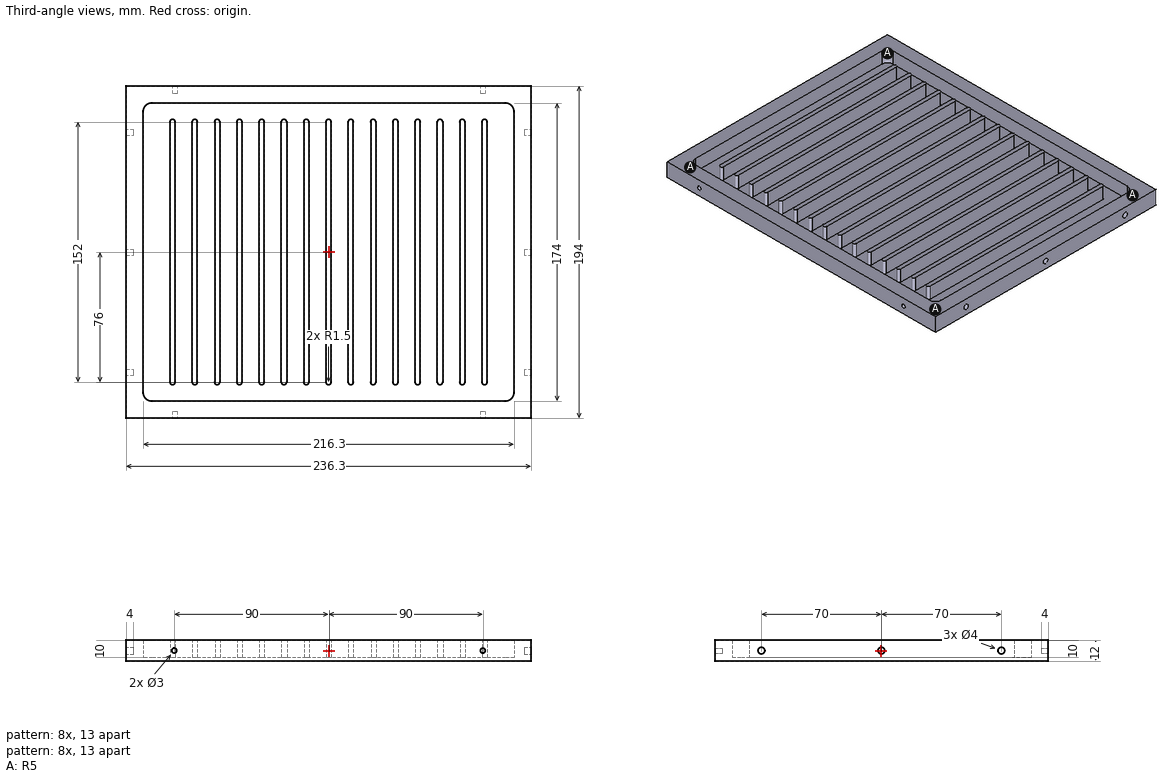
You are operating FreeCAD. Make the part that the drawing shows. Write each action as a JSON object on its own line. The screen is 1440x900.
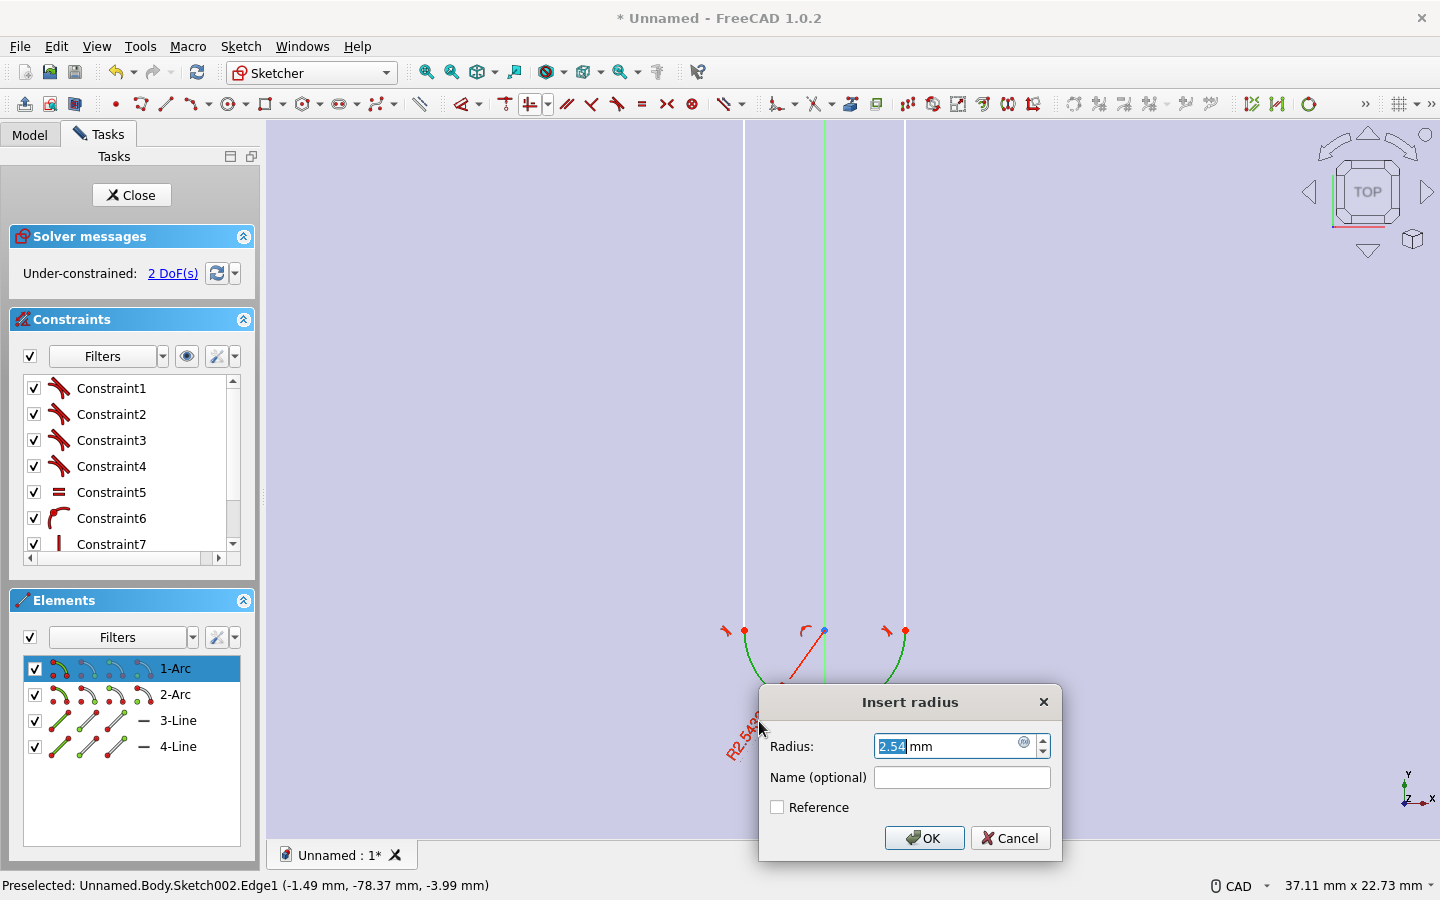
{"action": "type", "text": "1.5"}
{"action": "key", "text": "Return"}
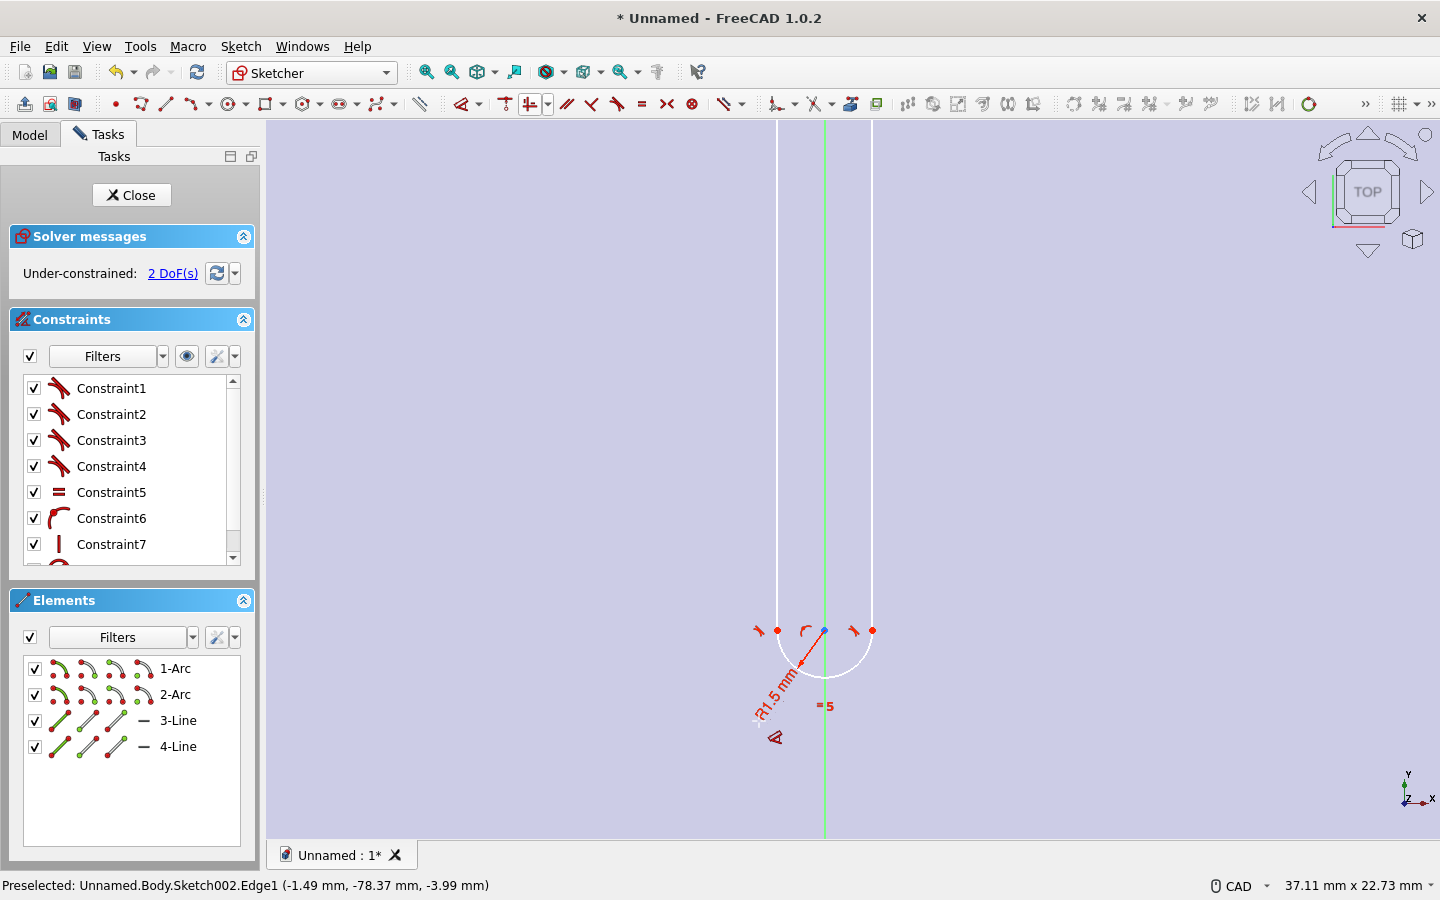
{"action": "scroll", "coordinate": [780, 705], "scroll_direction": "down", "scroll_amount": 12}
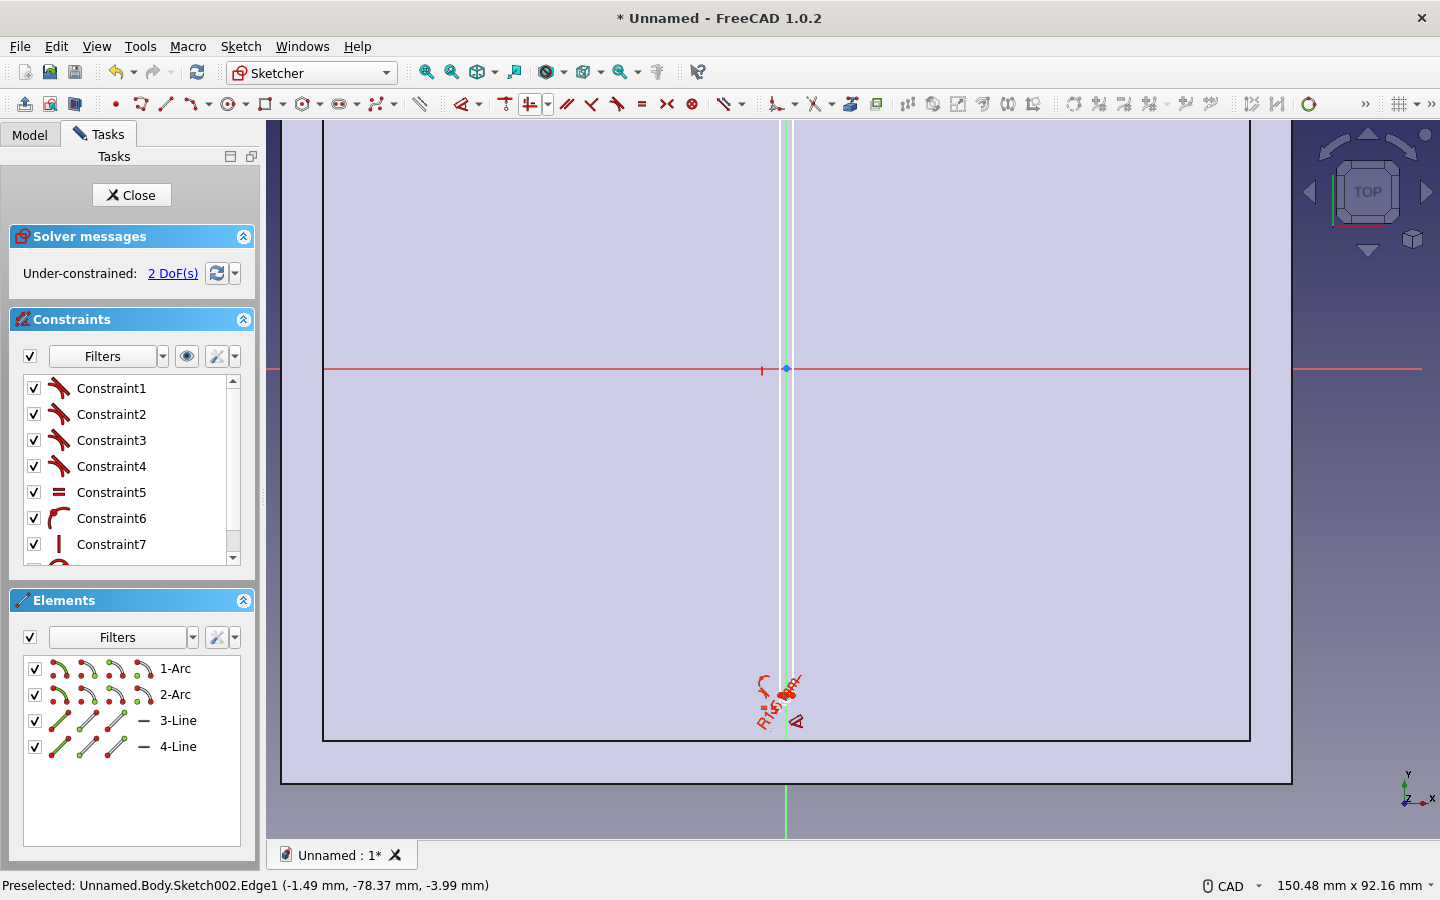
{"action": "scroll", "coordinate": [780, 568], "scroll_direction": "up", "scroll_amount": 6}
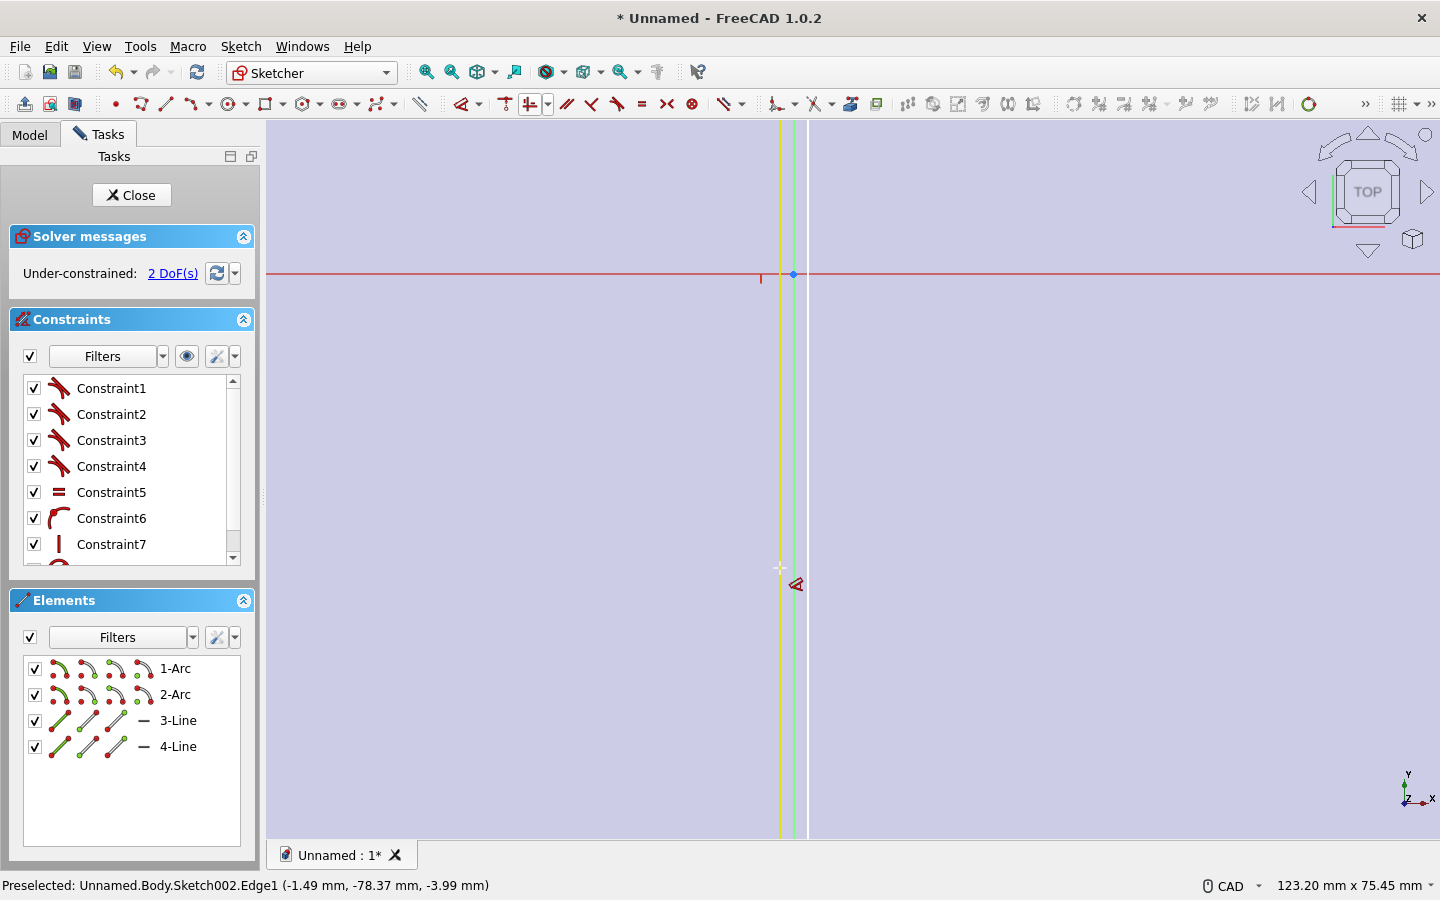
{"action": "left_click", "coordinate": [780, 567]}
{"action": "left_click", "coordinate": [746, 480]}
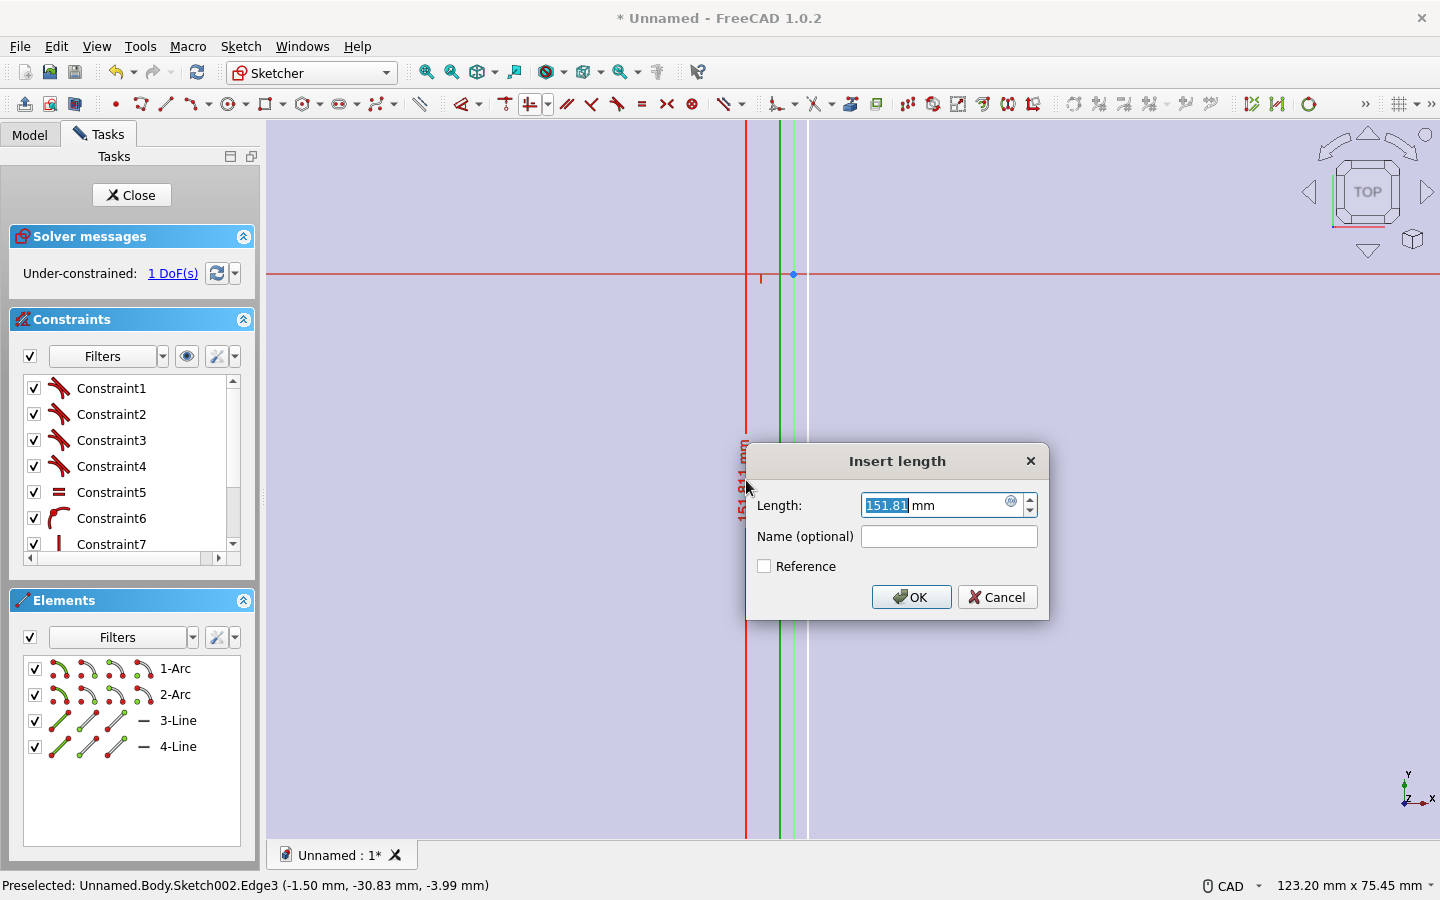
{"action": "type", "text": "152"}
{"action": "key", "text": "Return"}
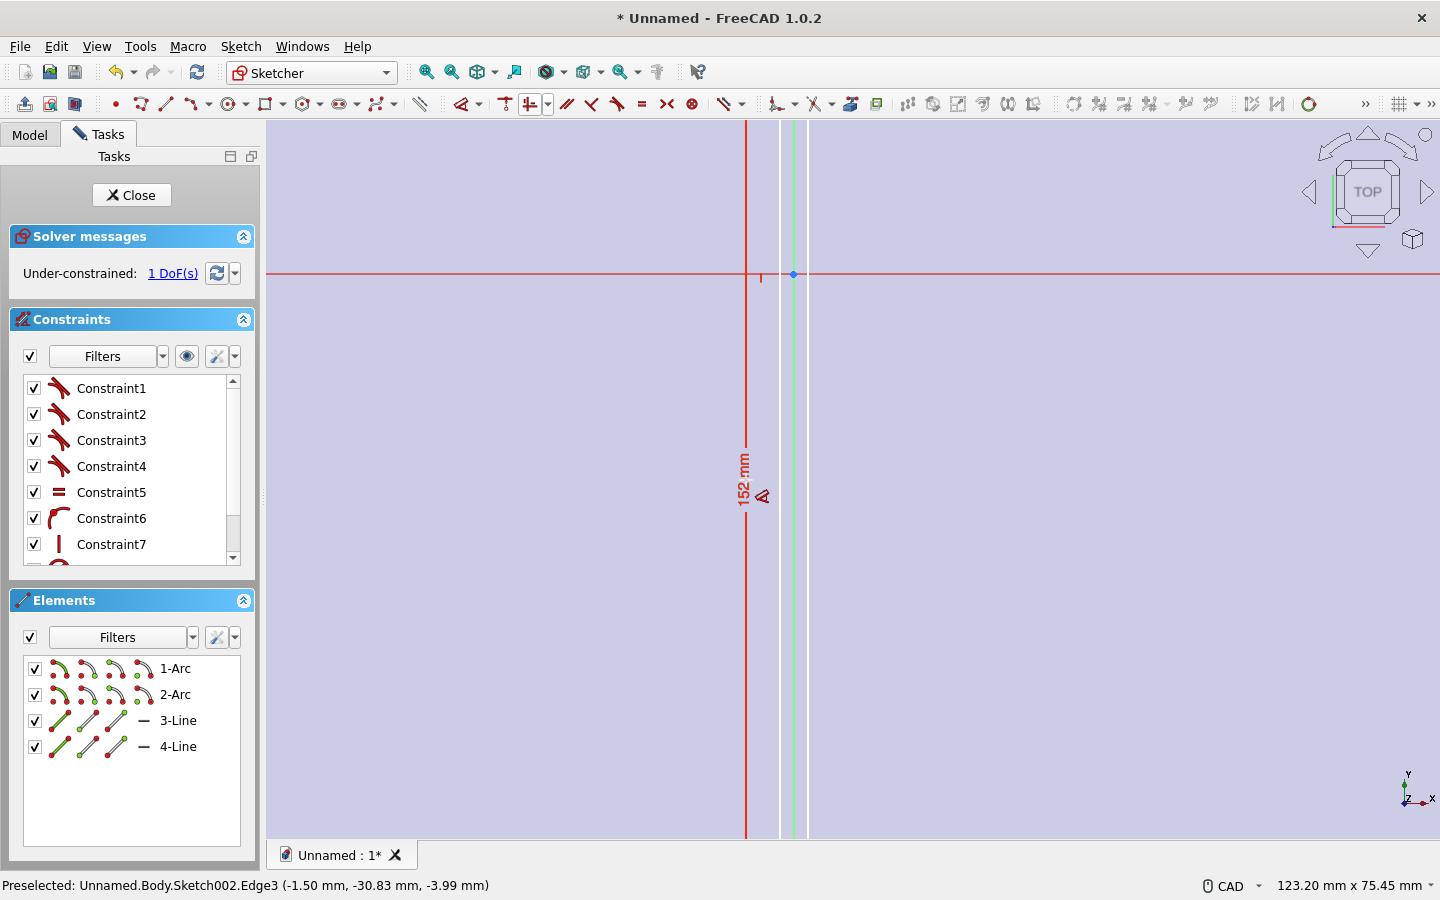
{"action": "scroll", "coordinate": [780, 568], "scroll_direction": "down", "scroll_amount": 6}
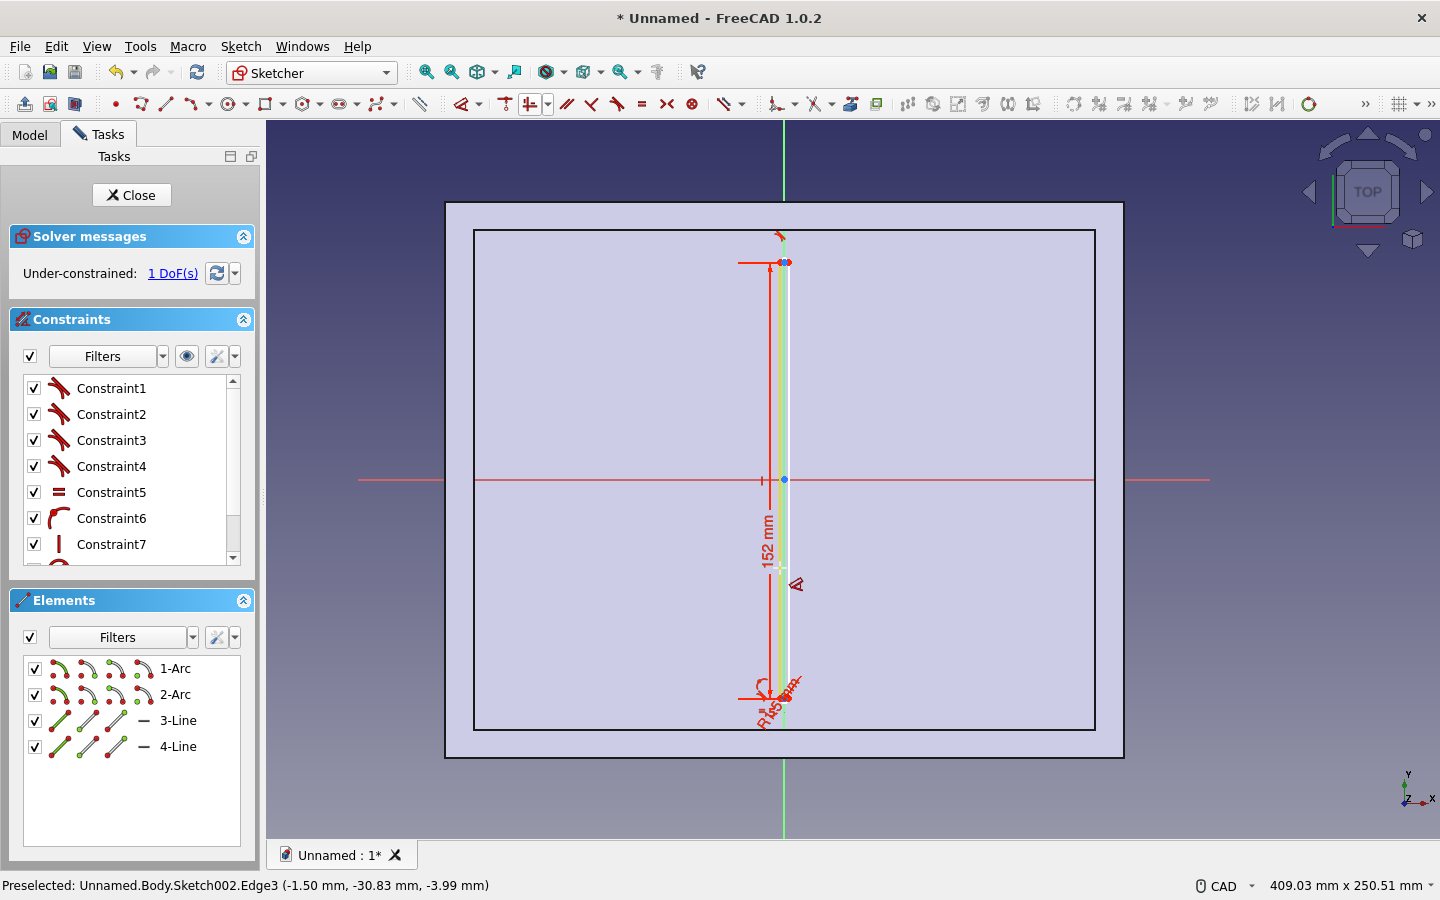
{"action": "scroll", "coordinate": [780, 699], "scroll_direction": "up", "scroll_amount": 6}